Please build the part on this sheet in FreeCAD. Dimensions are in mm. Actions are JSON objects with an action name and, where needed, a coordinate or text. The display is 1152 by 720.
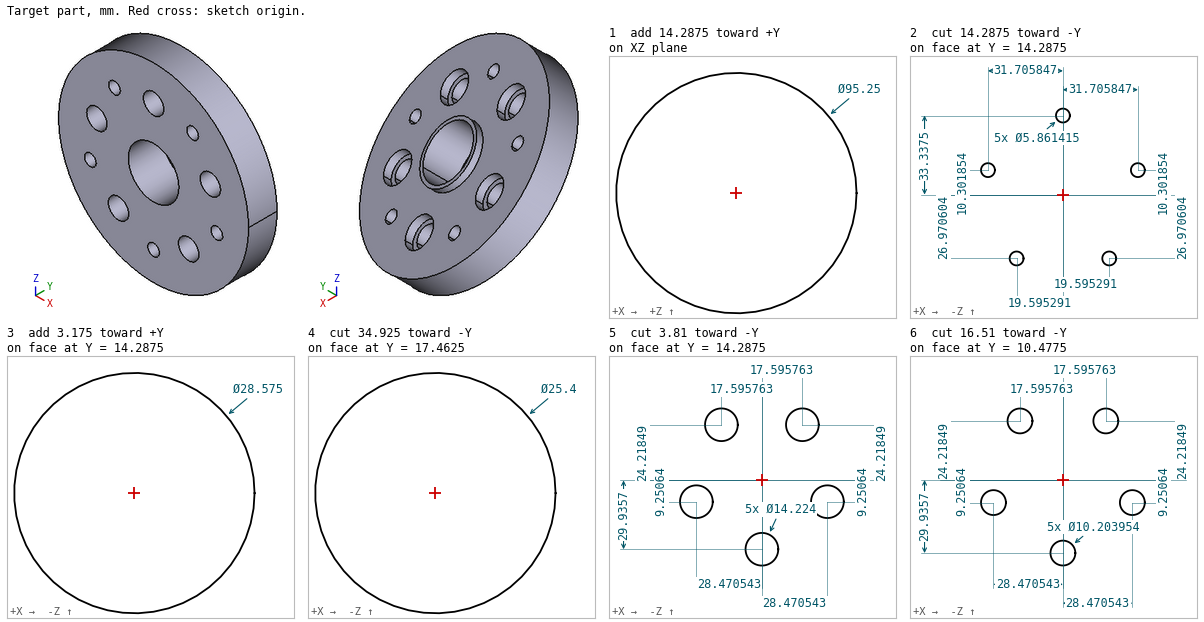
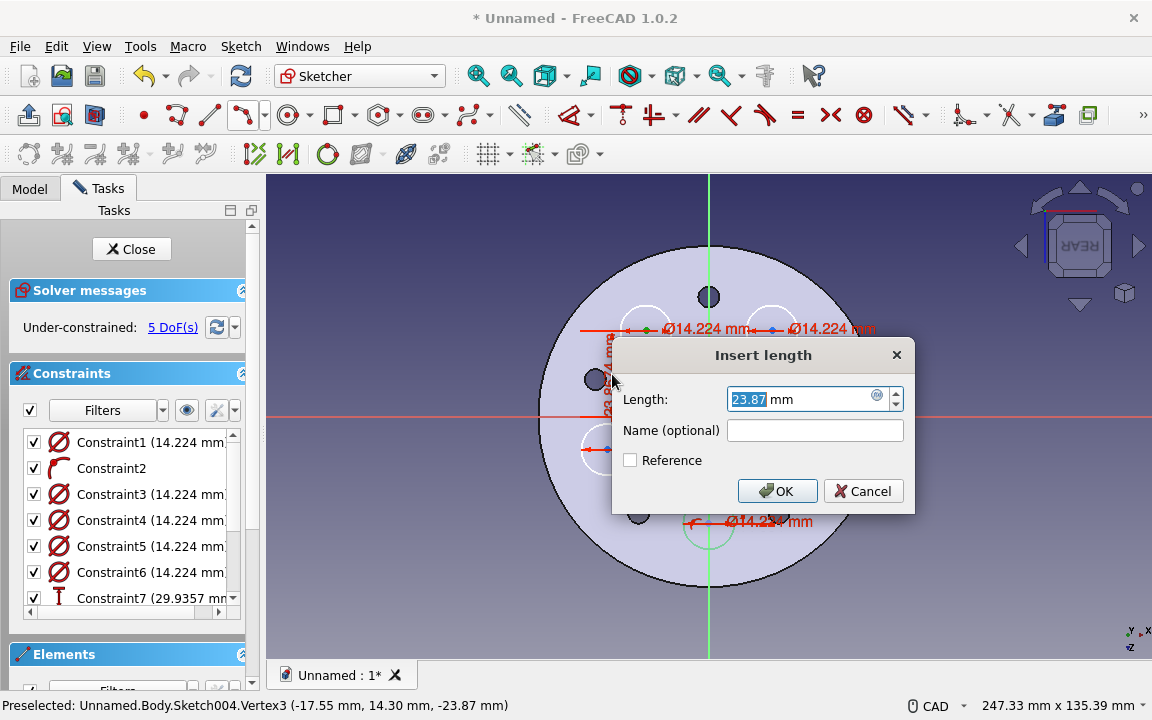
{"action": "type", "text": "24.21849"}
{"action": "key", "text": "Return"}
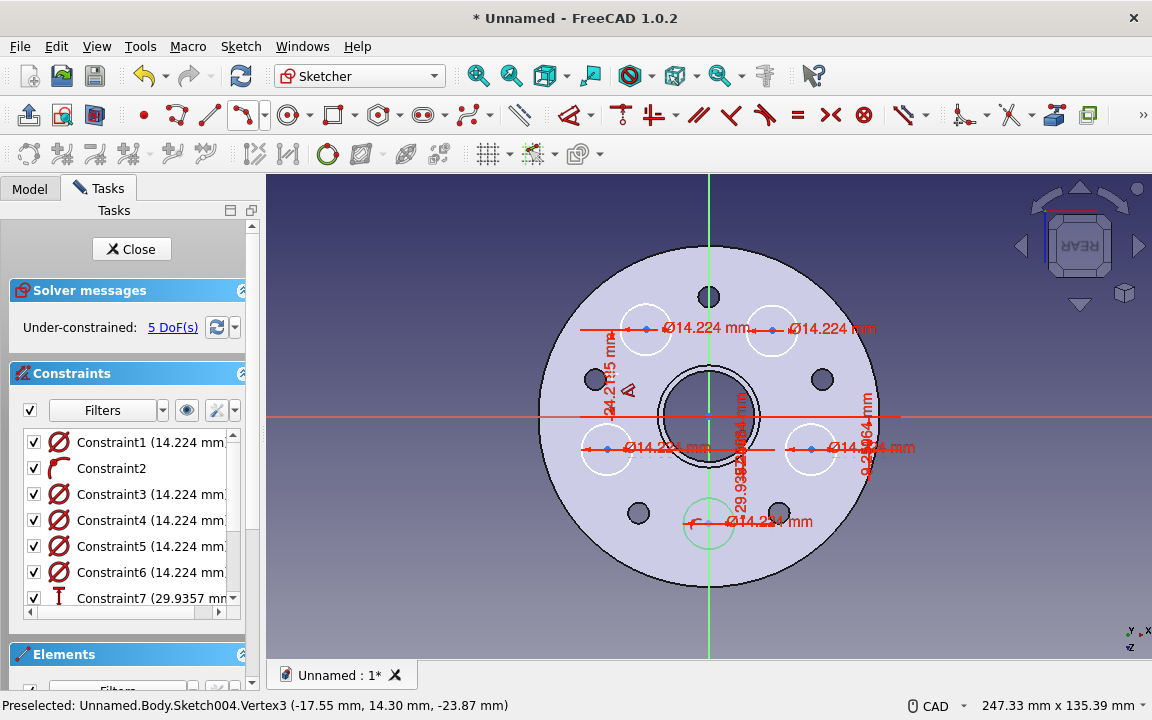
{"action": "left_click", "coordinate": [772, 331]}
{"action": "left_click", "coordinate": [806, 374]}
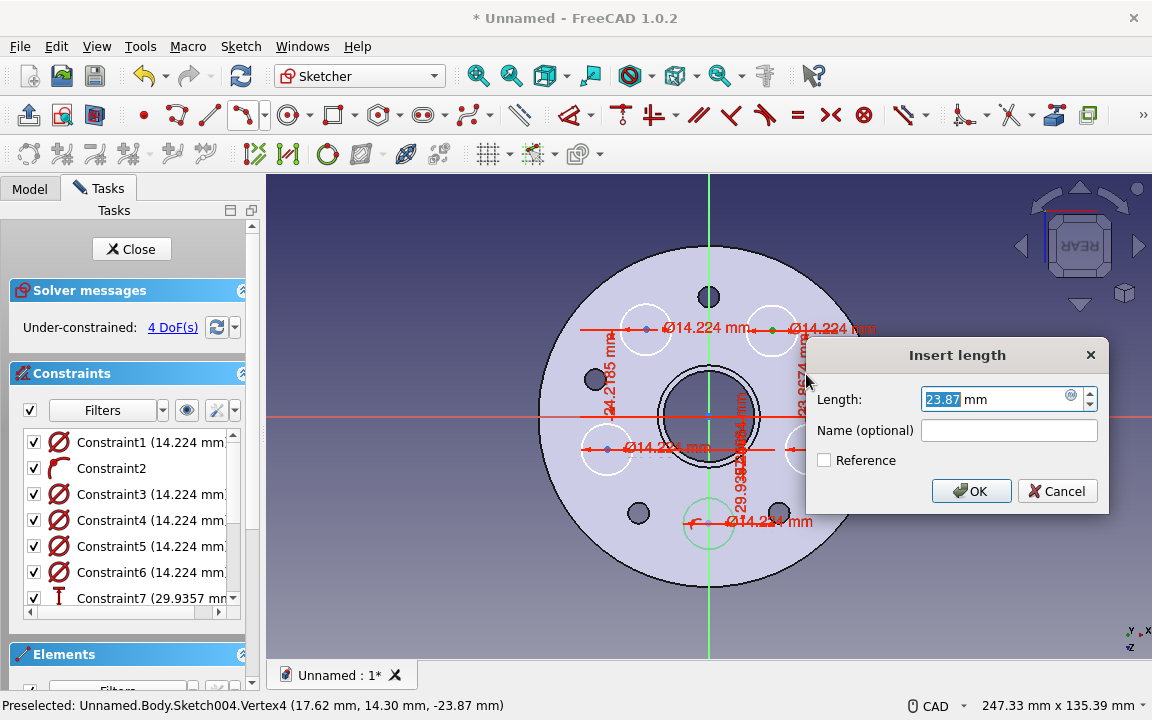
{"action": "type", "text": "24.21849"}
{"action": "key", "text": "Return"}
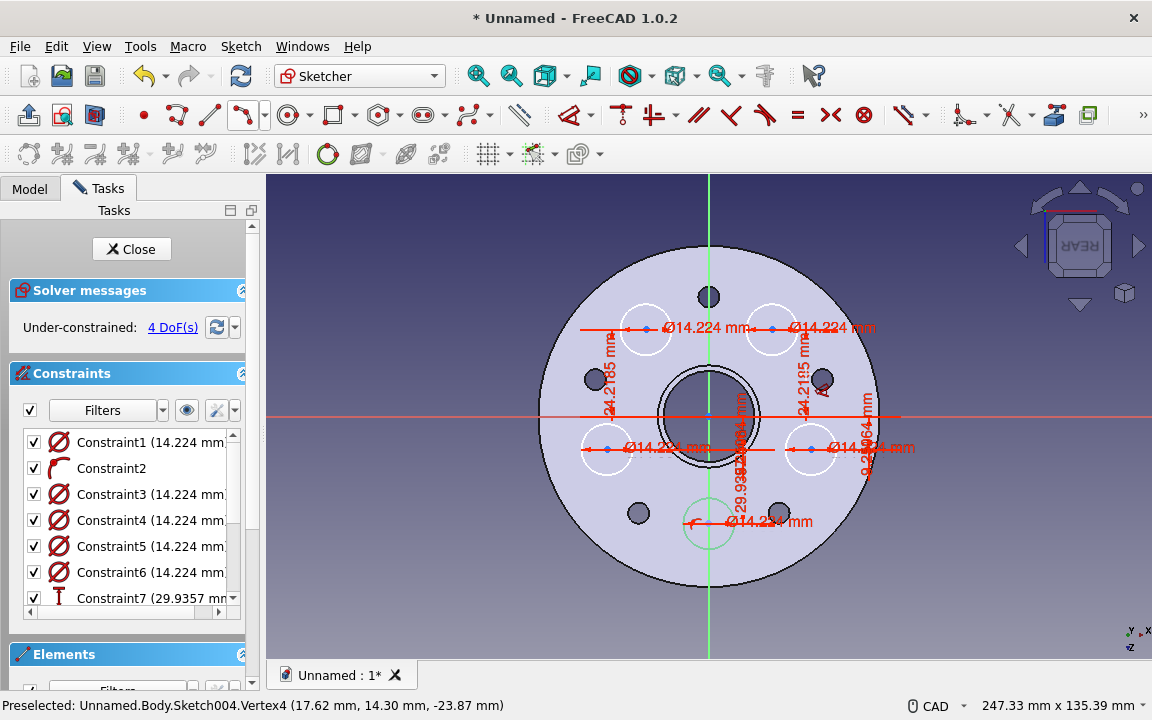
{"action": "left_click", "coordinate": [607, 450]}
{"action": "left_click", "coordinate": [658, 484]}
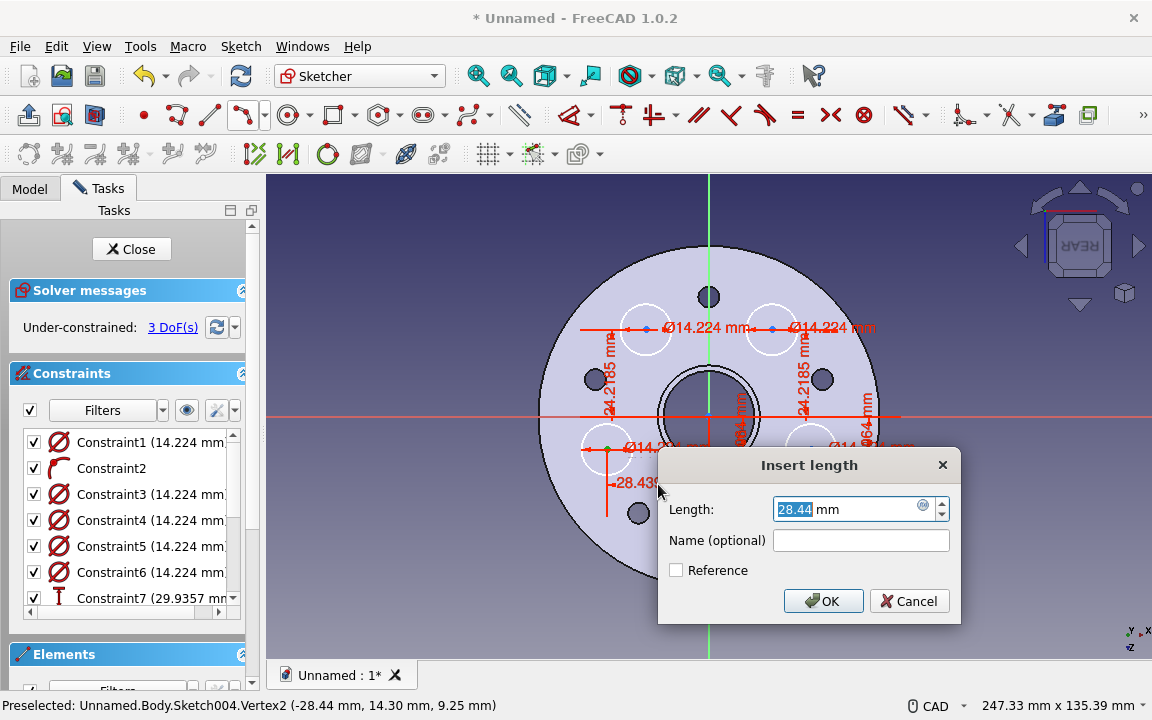
{"action": "type", "text": "28.470543"}
{"action": "key", "text": "Return"}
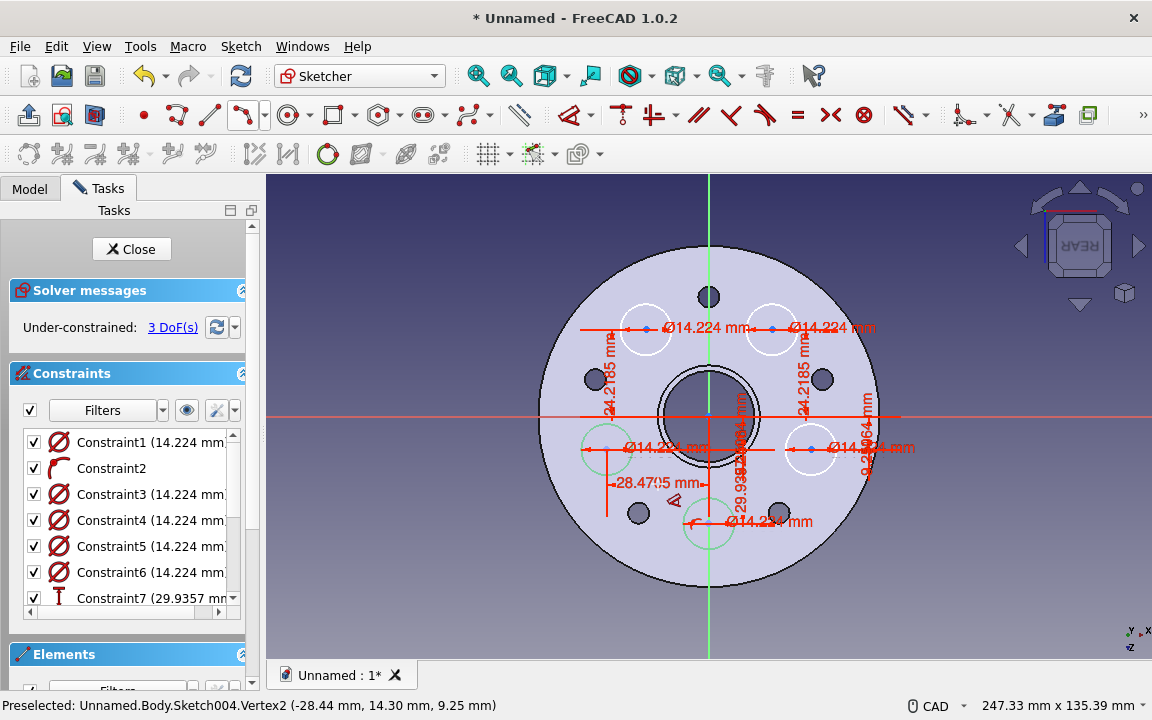
{"action": "left_click", "coordinate": [646, 330]}
{"action": "left_click", "coordinate": [677, 296]}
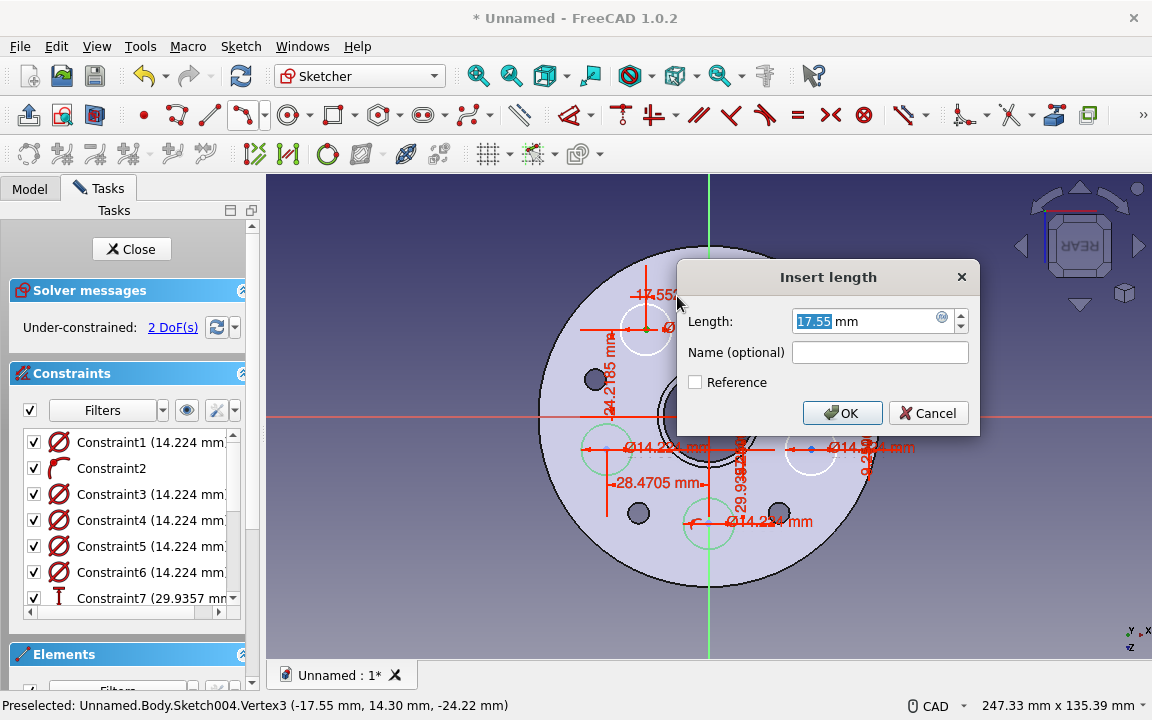
{"action": "type", "text": "17.595763"}
{"action": "key", "text": "Return"}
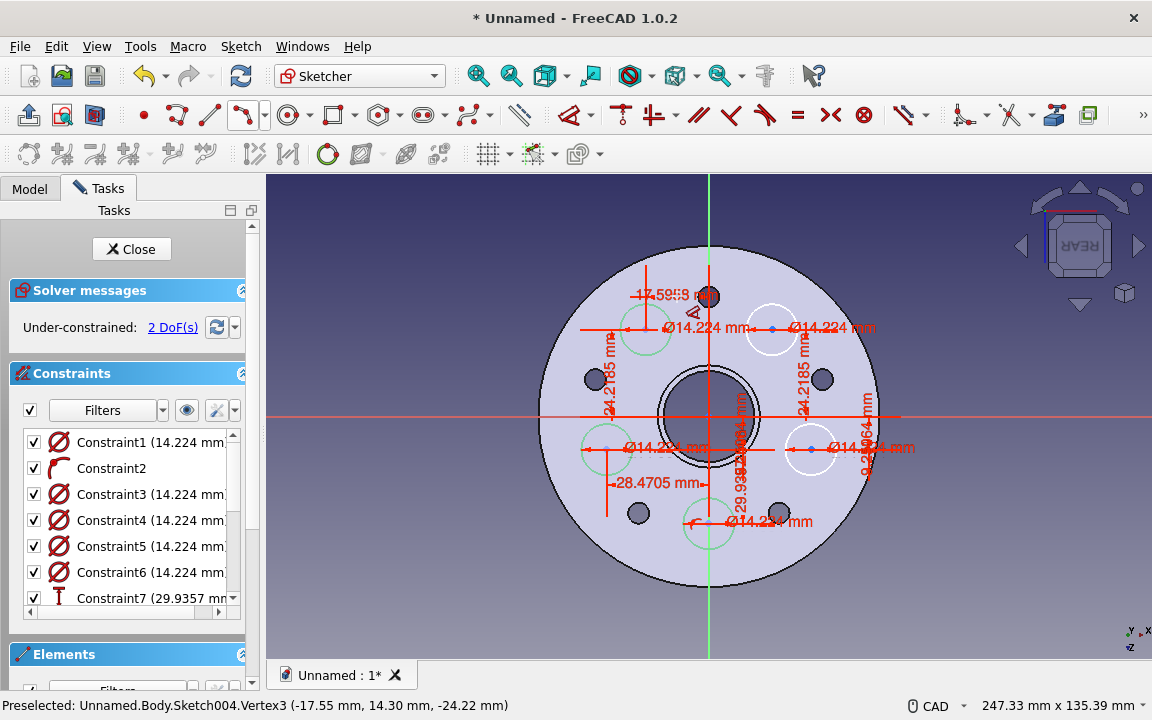
{"action": "left_click", "coordinate": [772, 330]}
{"action": "left_click", "coordinate": [740, 272]}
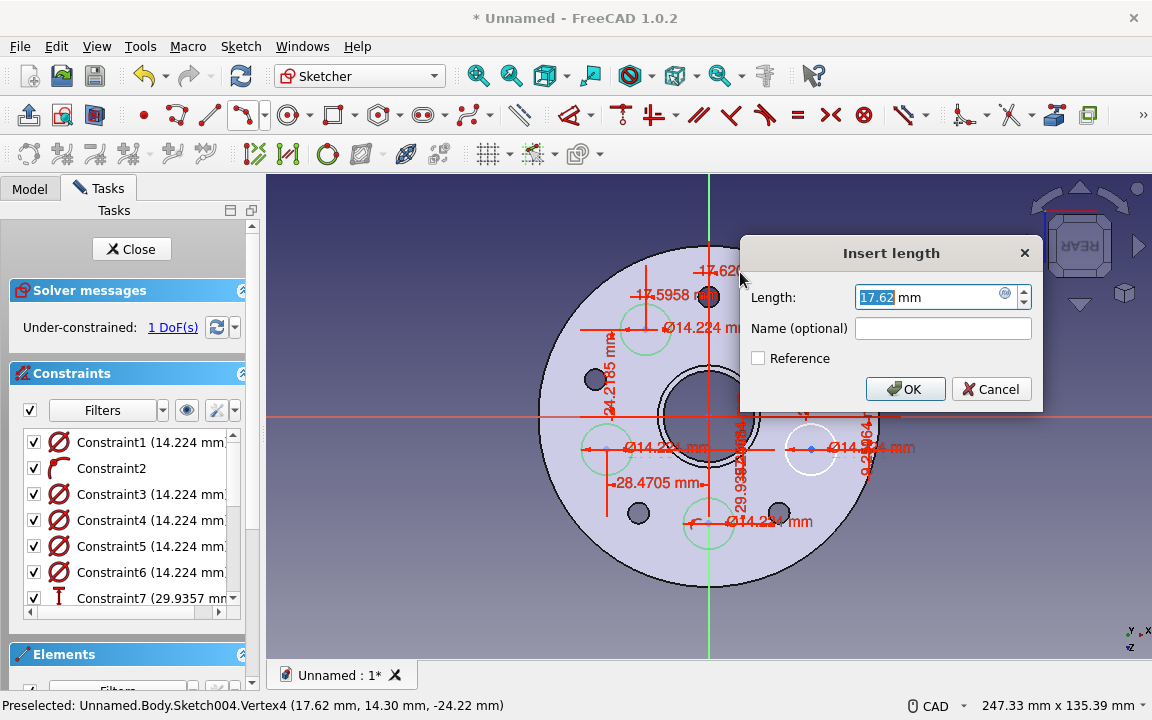
{"action": "type", "text": "17.595763"}
{"action": "key", "text": "Return"}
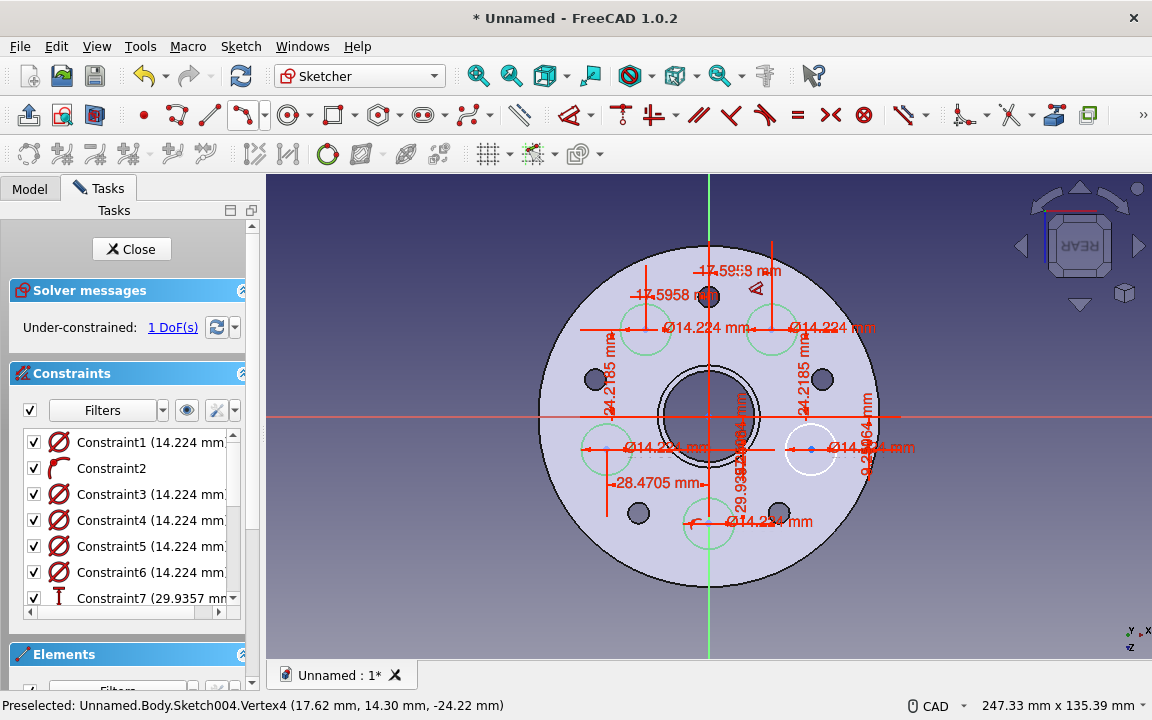
{"action": "left_click", "coordinate": [811, 450]}
{"action": "left_click", "coordinate": [724, 382]}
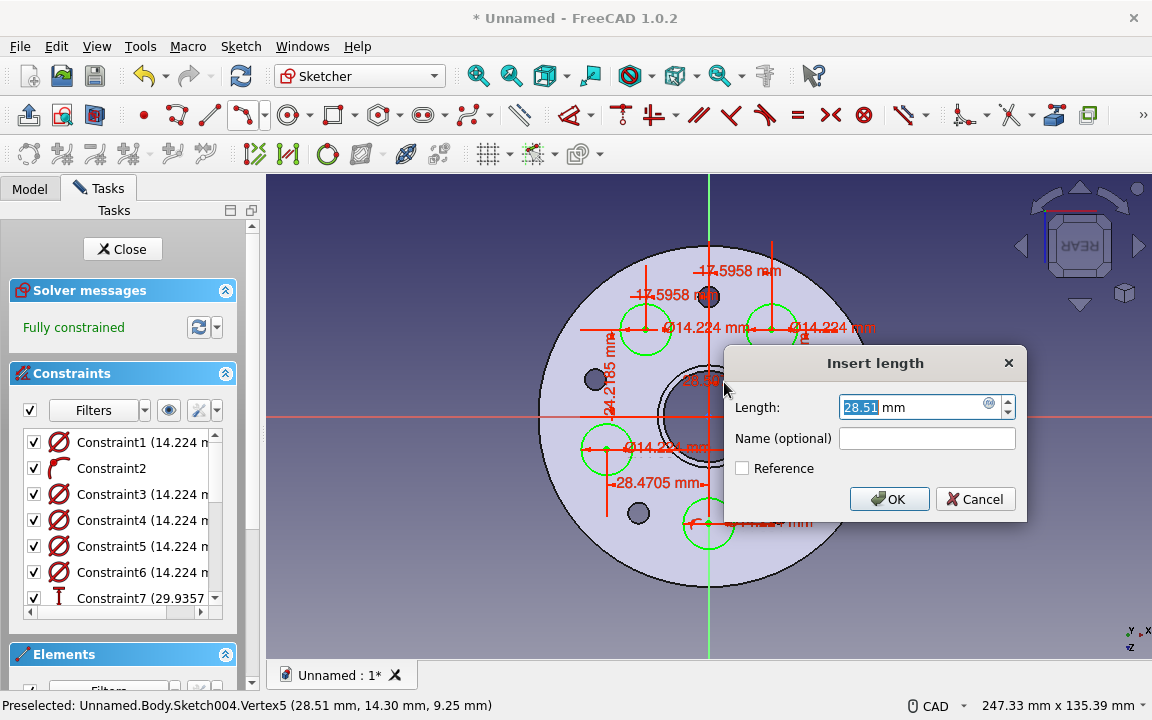
{"action": "type", "text": "28.470543"}
{"action": "key", "text": "Return"}
{"action": "key", "text": "Escape"}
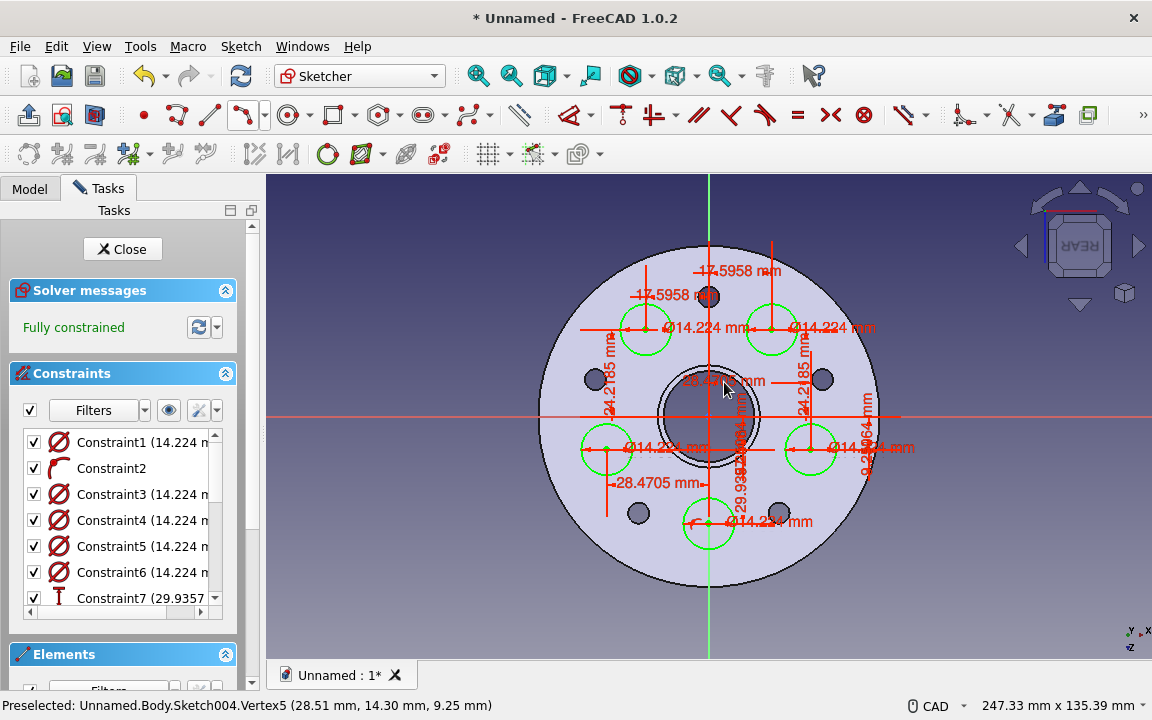
{"action": "left_click", "coordinate": [123, 249]}